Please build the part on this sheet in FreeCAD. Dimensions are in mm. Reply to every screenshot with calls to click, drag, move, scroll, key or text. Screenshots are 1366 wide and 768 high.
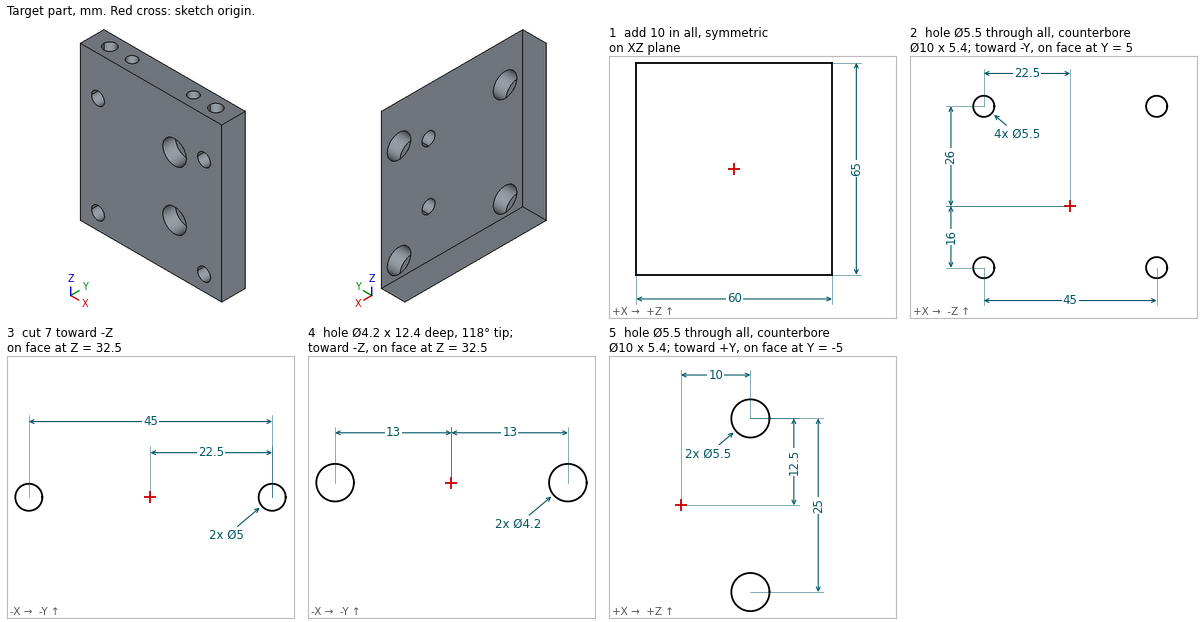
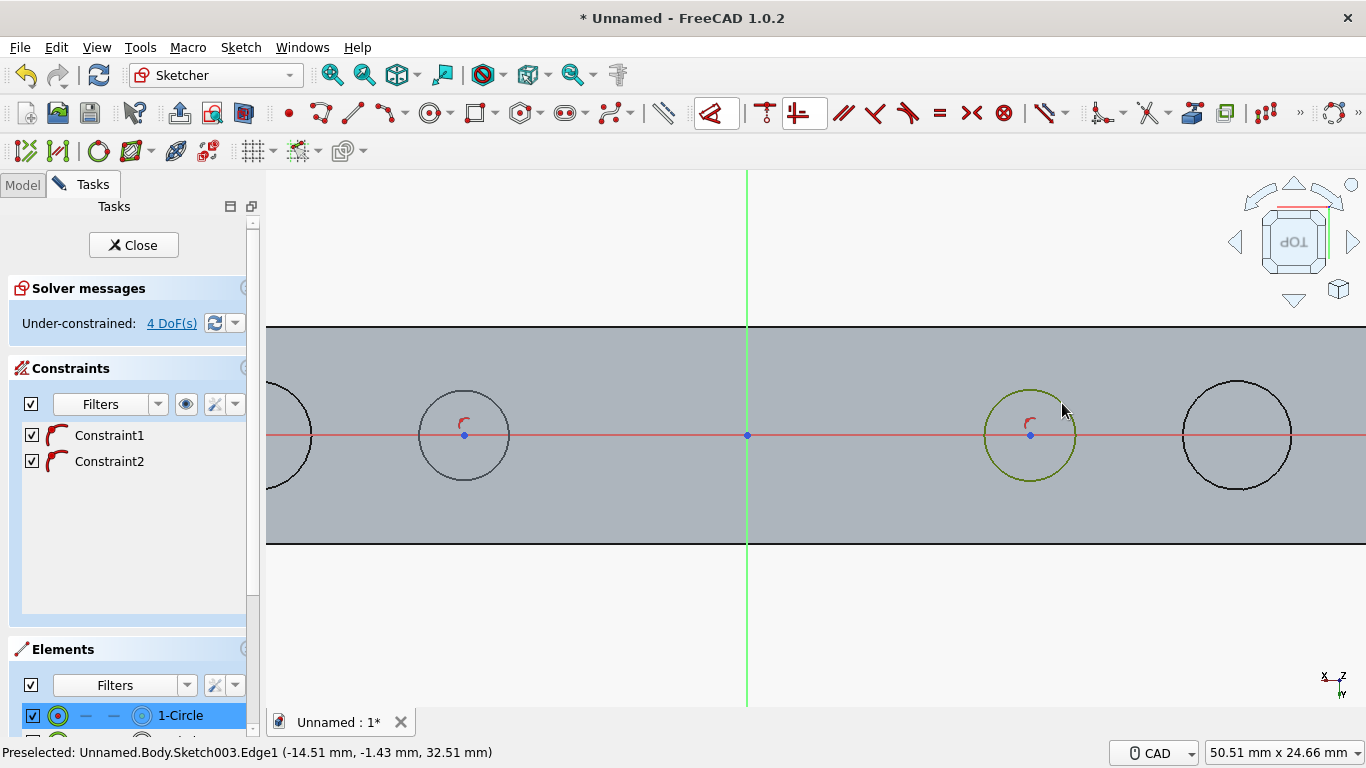
click(496, 404)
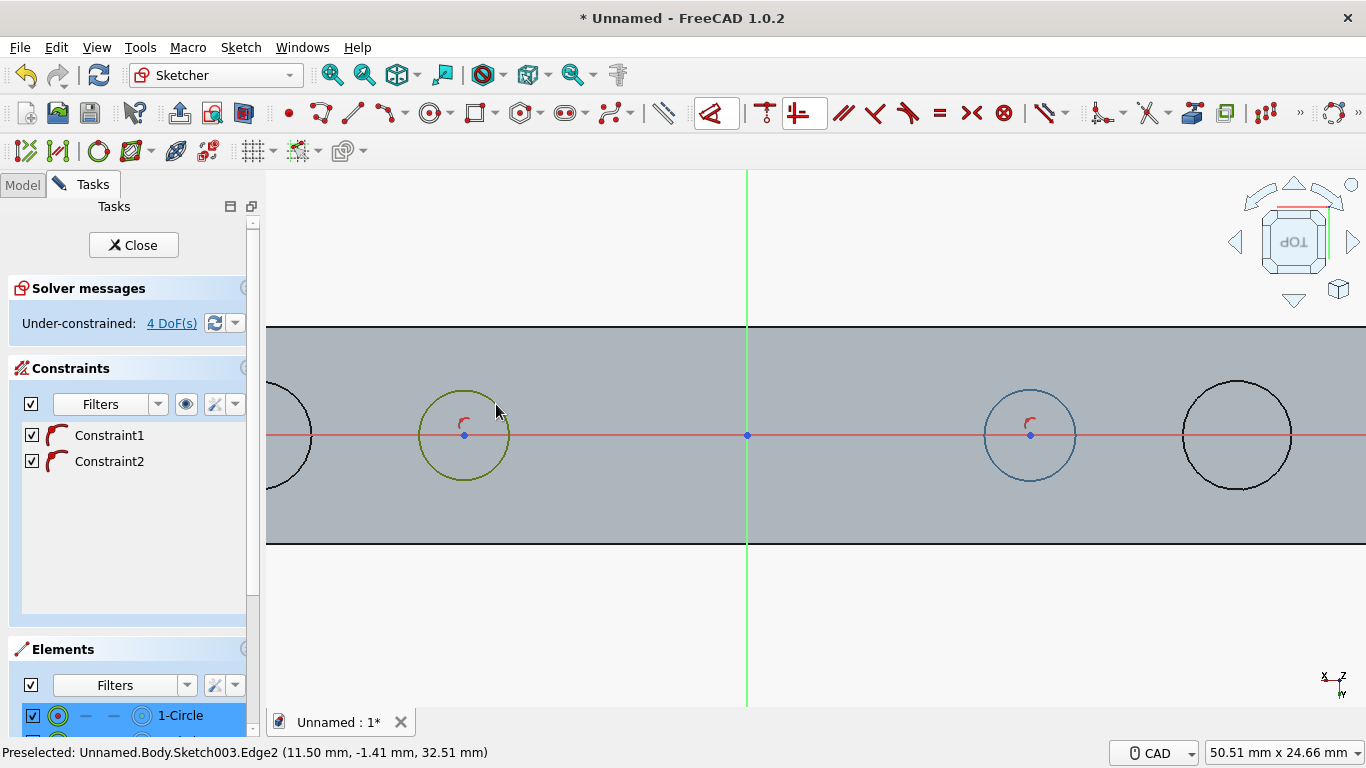
key(e)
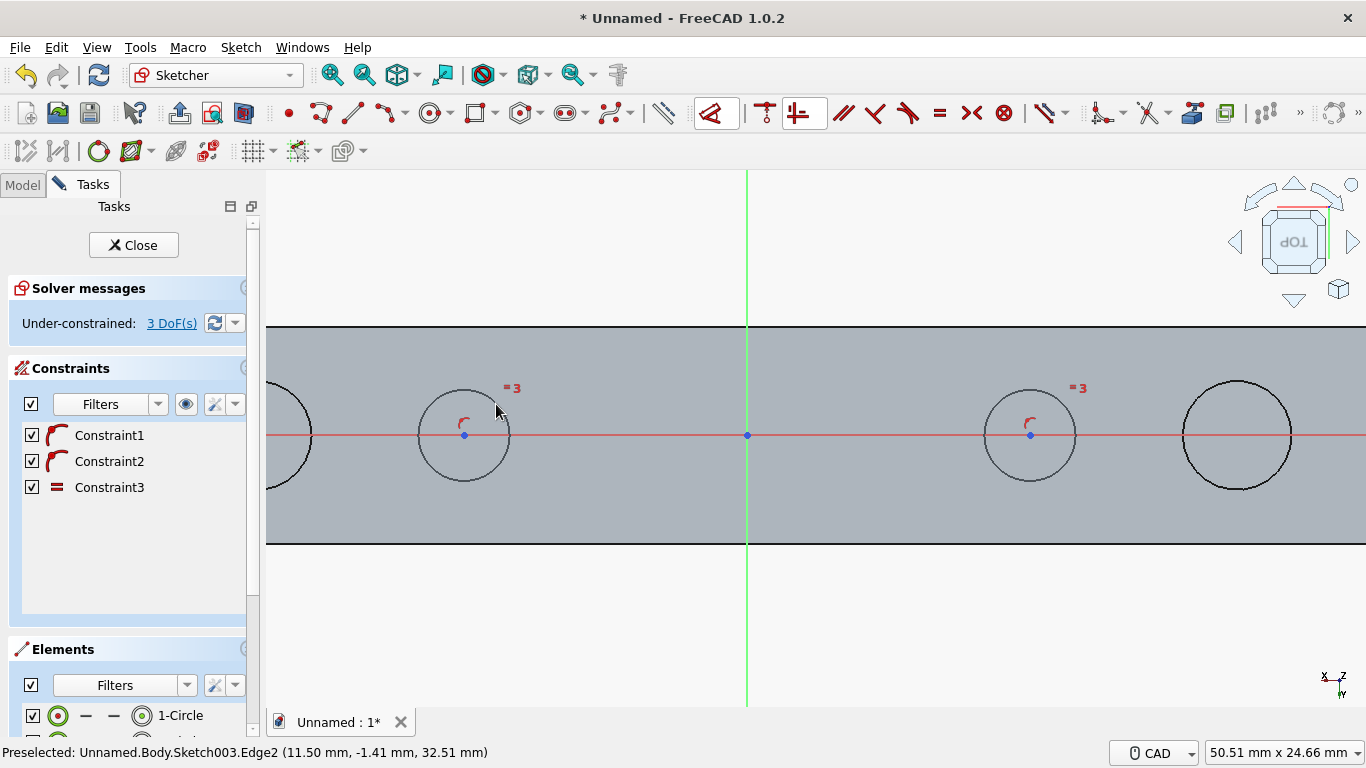
click(1062, 403)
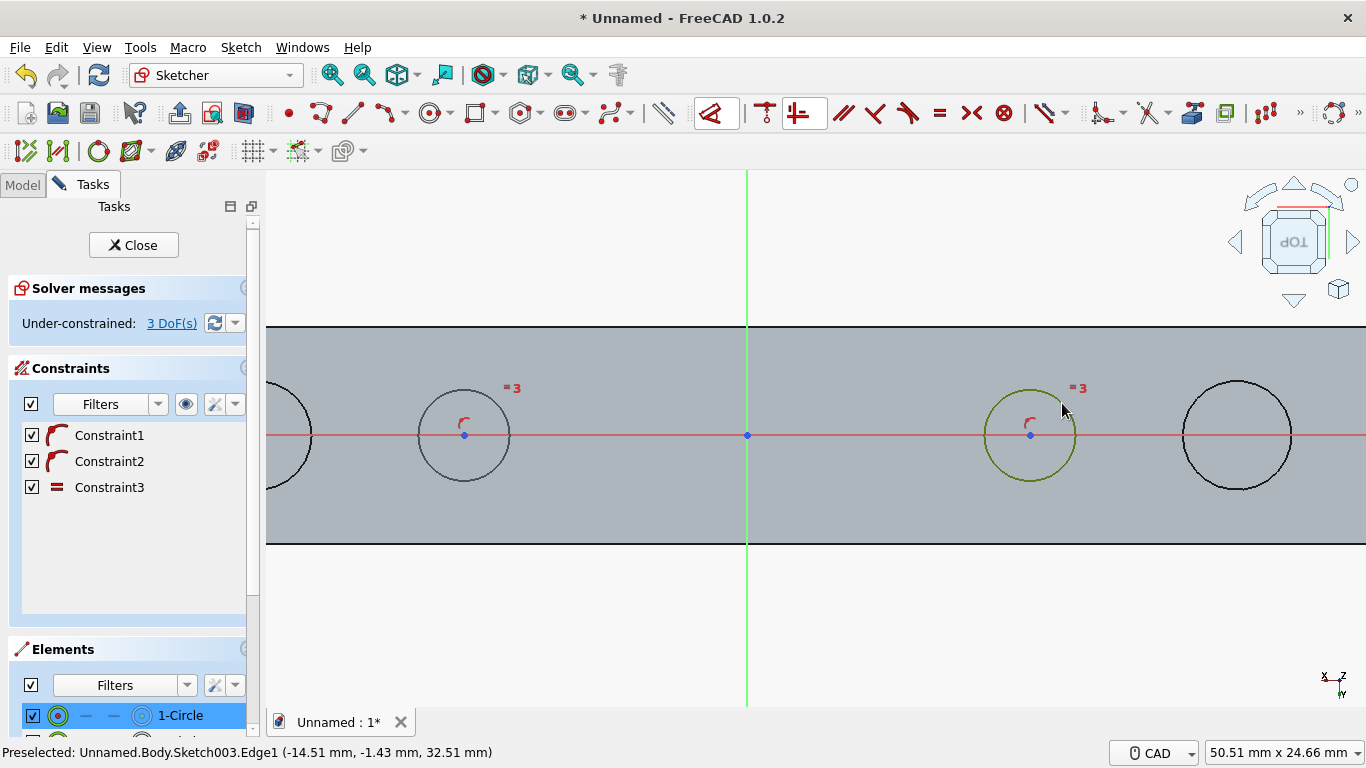
key(k)
key(o)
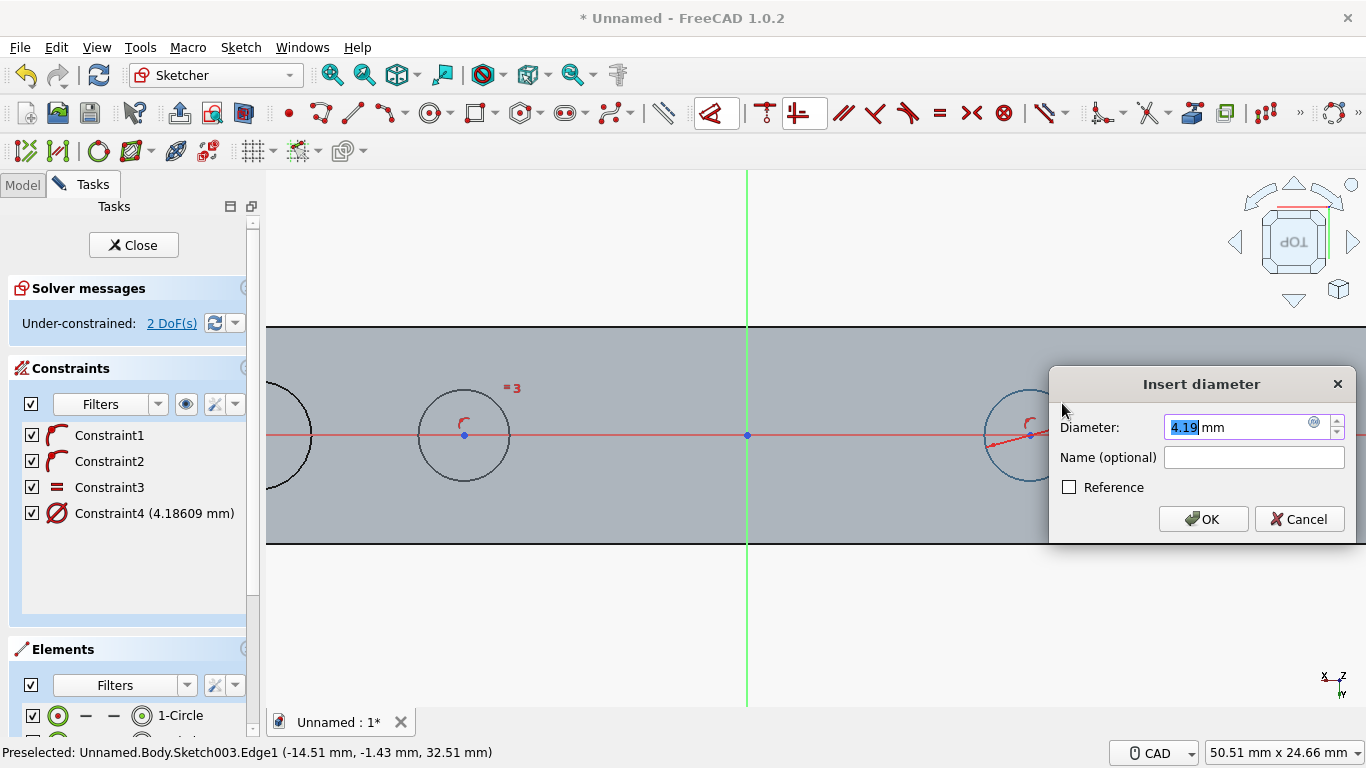
text(4.2)
key(Return)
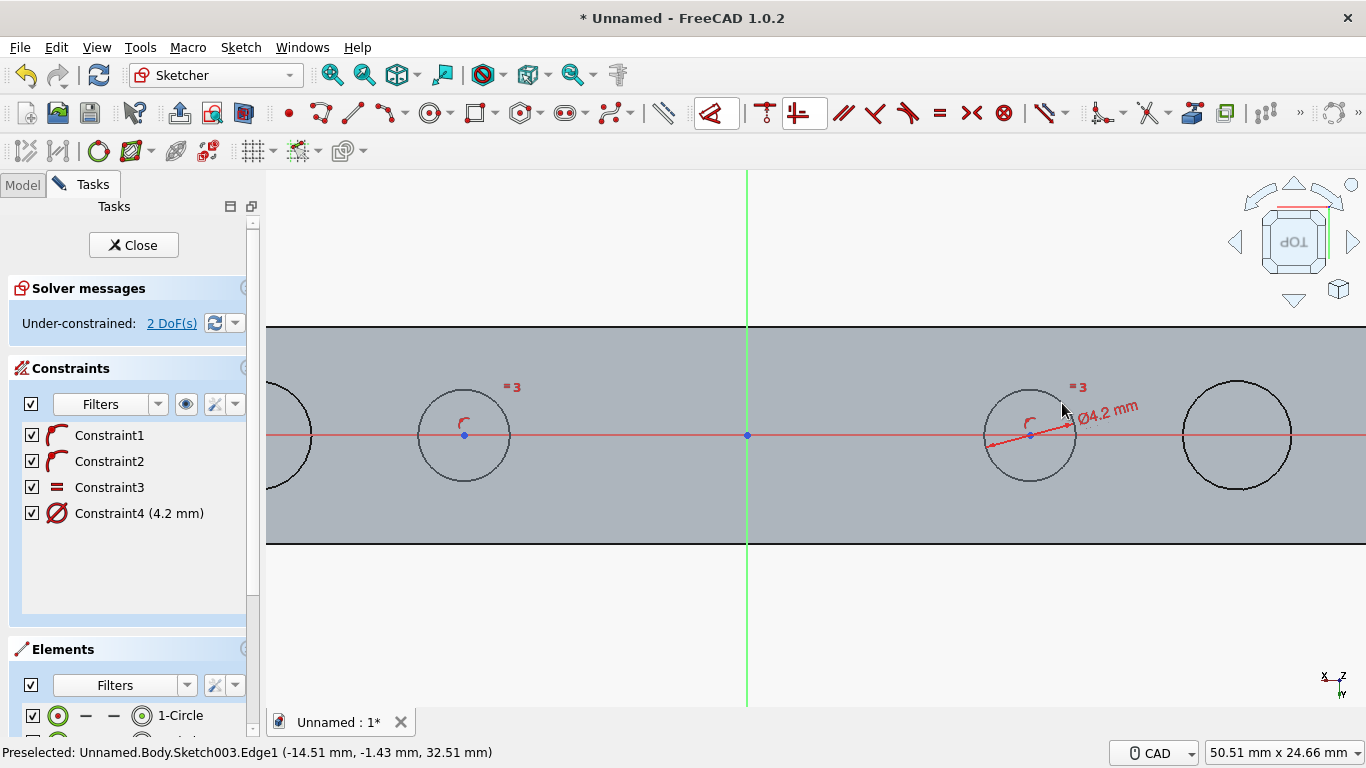
click(1030, 435)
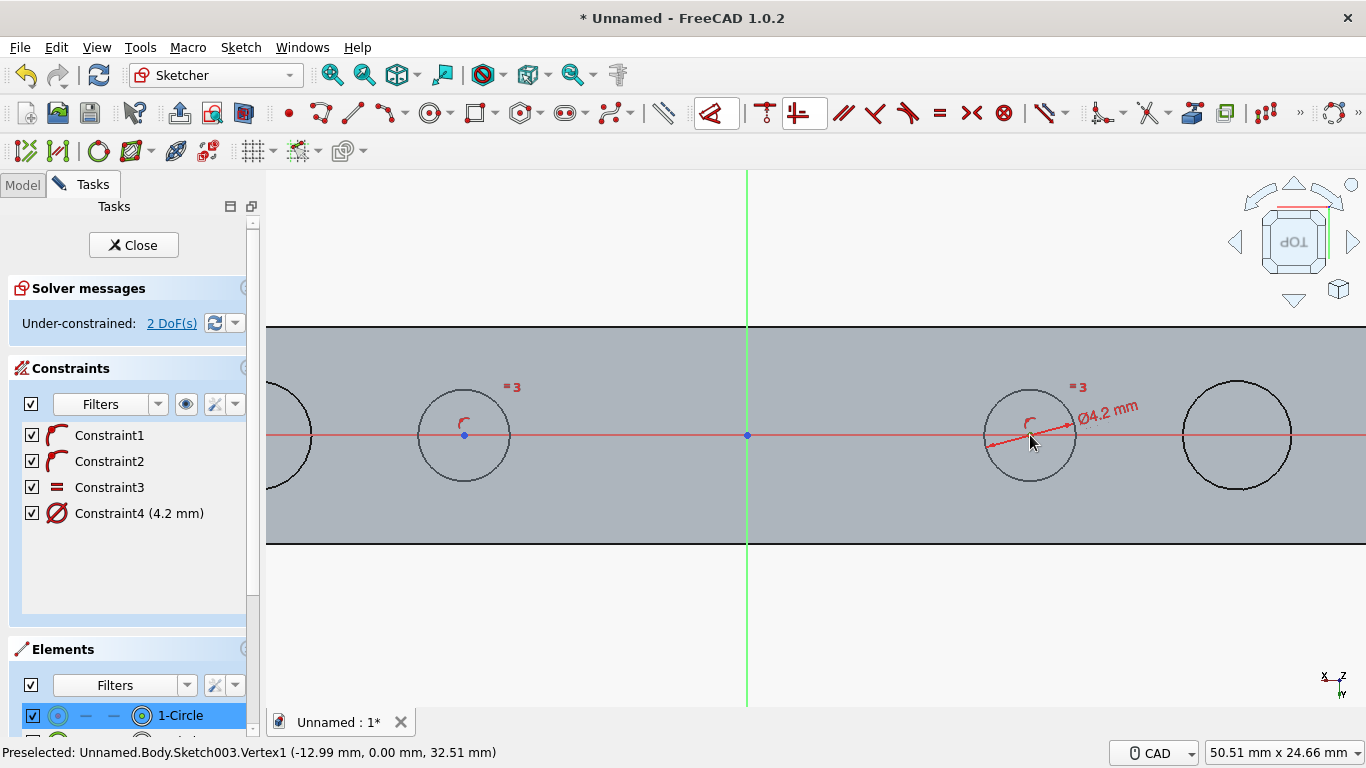
click(734, 114)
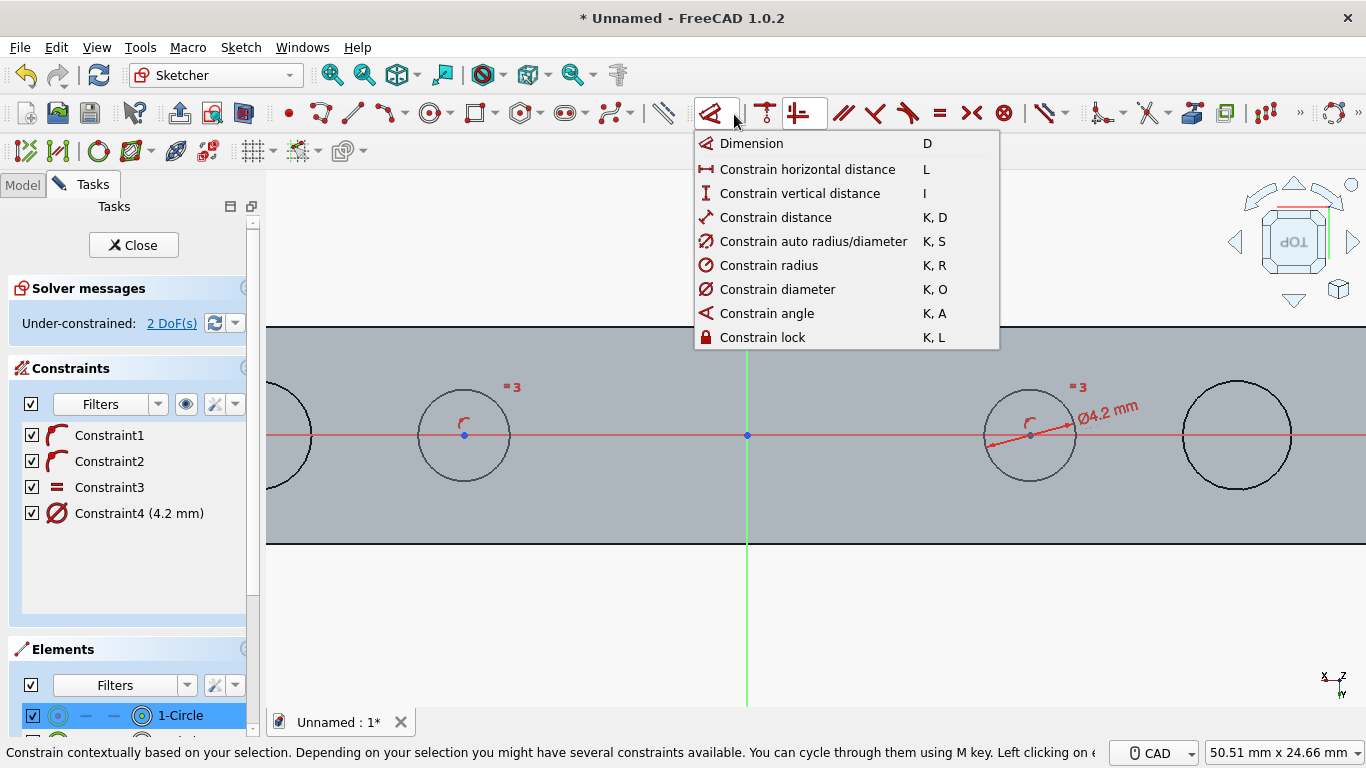
click(847, 169)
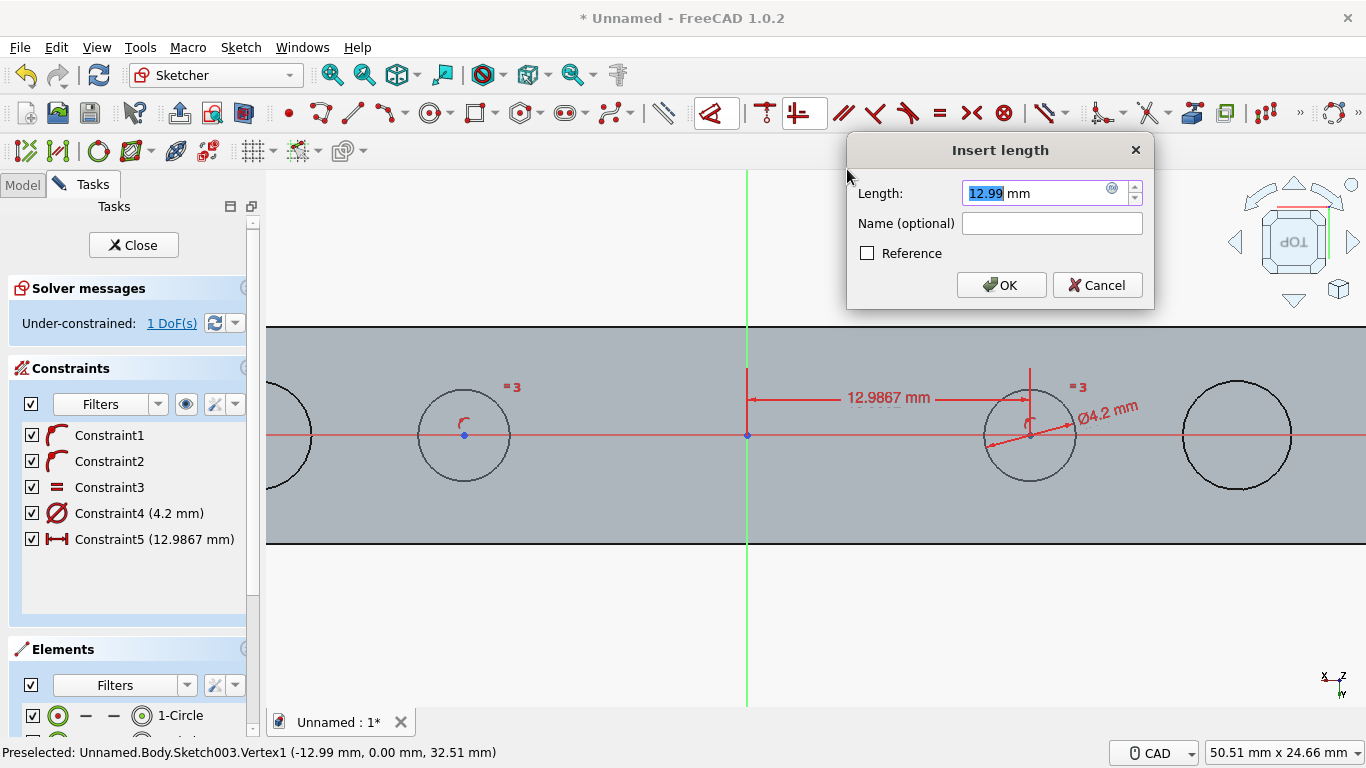
text(13)
key(Return)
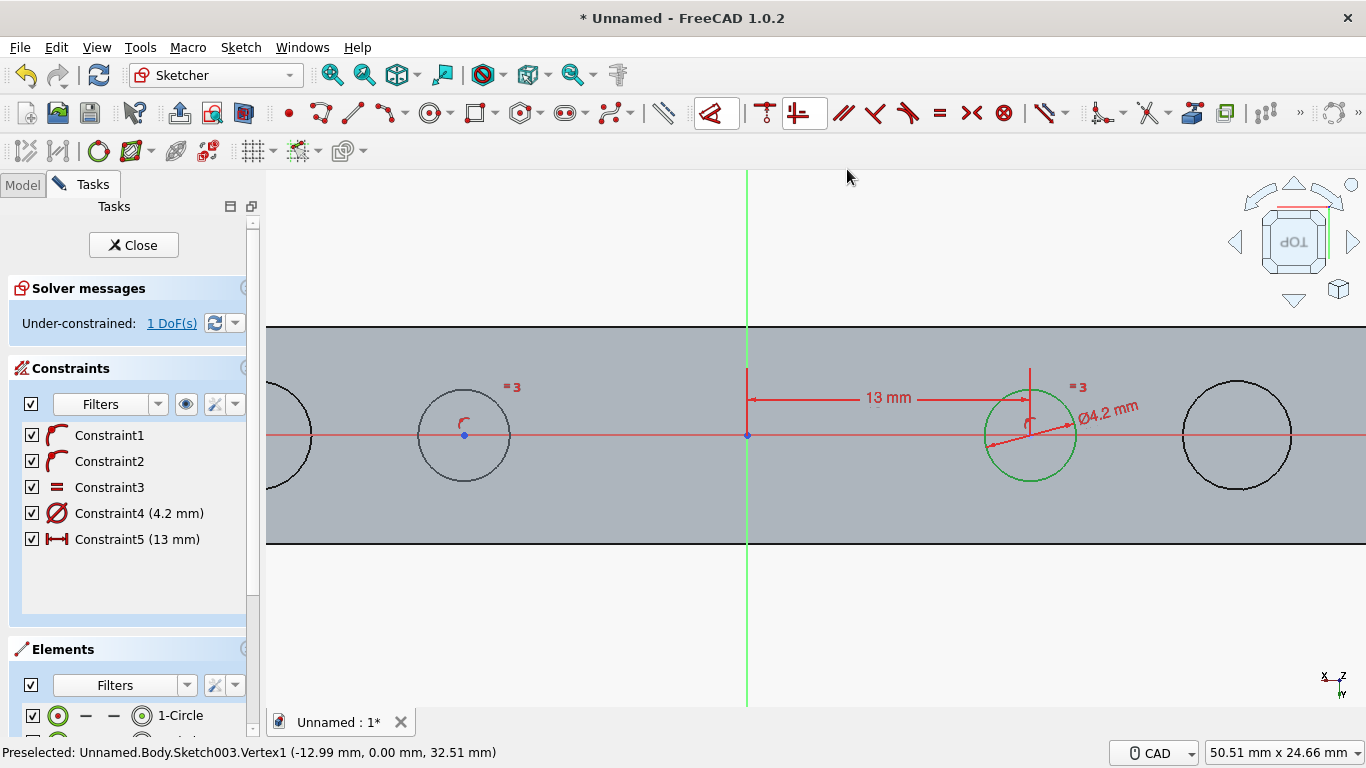
click(464, 435)